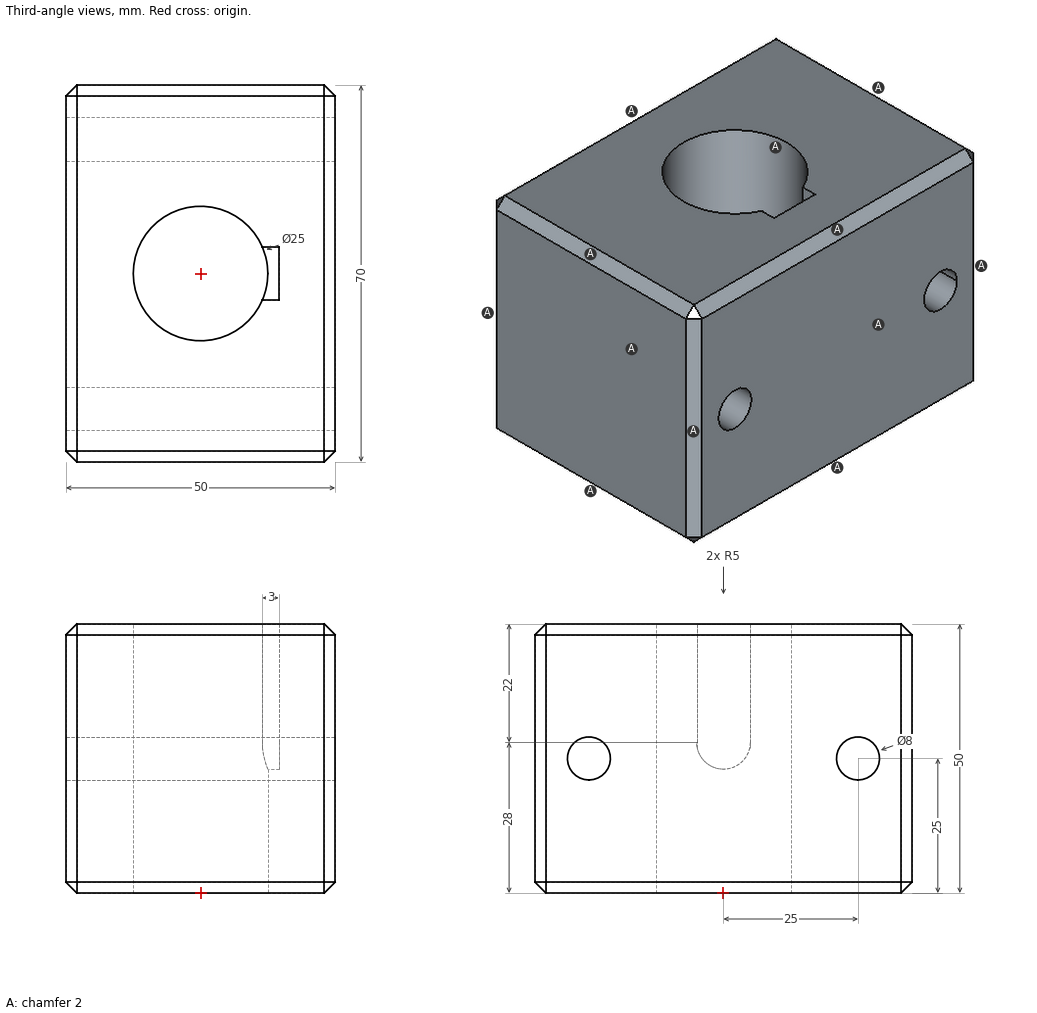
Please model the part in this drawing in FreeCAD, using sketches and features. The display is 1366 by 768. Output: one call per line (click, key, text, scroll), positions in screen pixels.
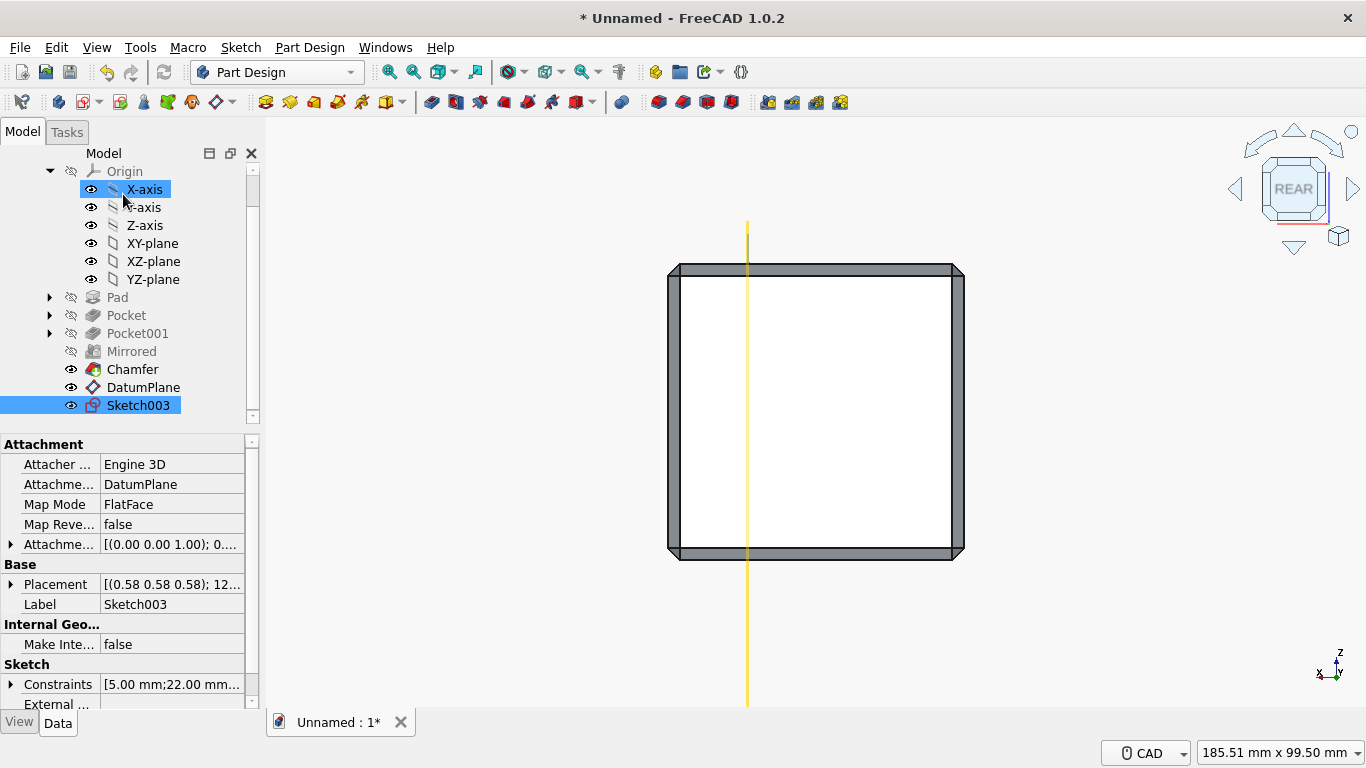
click(432, 102)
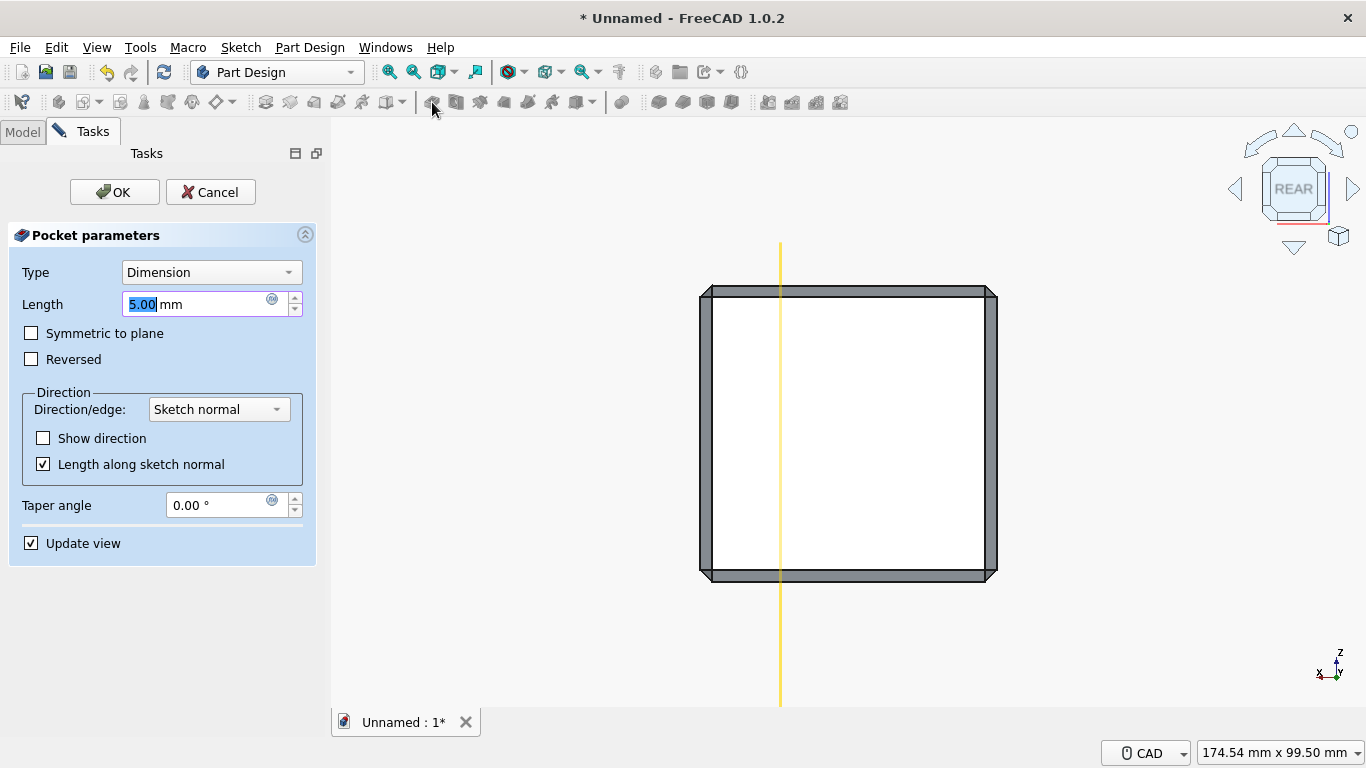
text(3)
key(Tab)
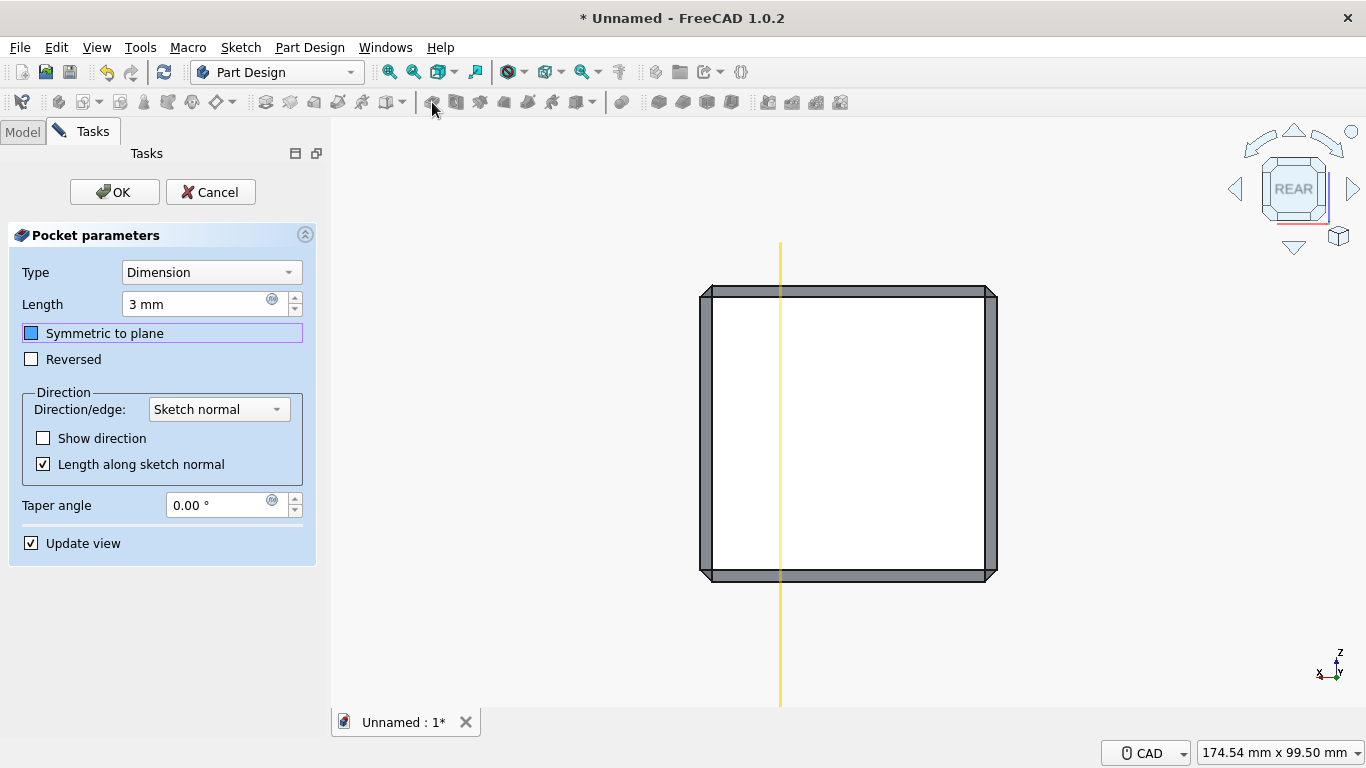
click(30, 359)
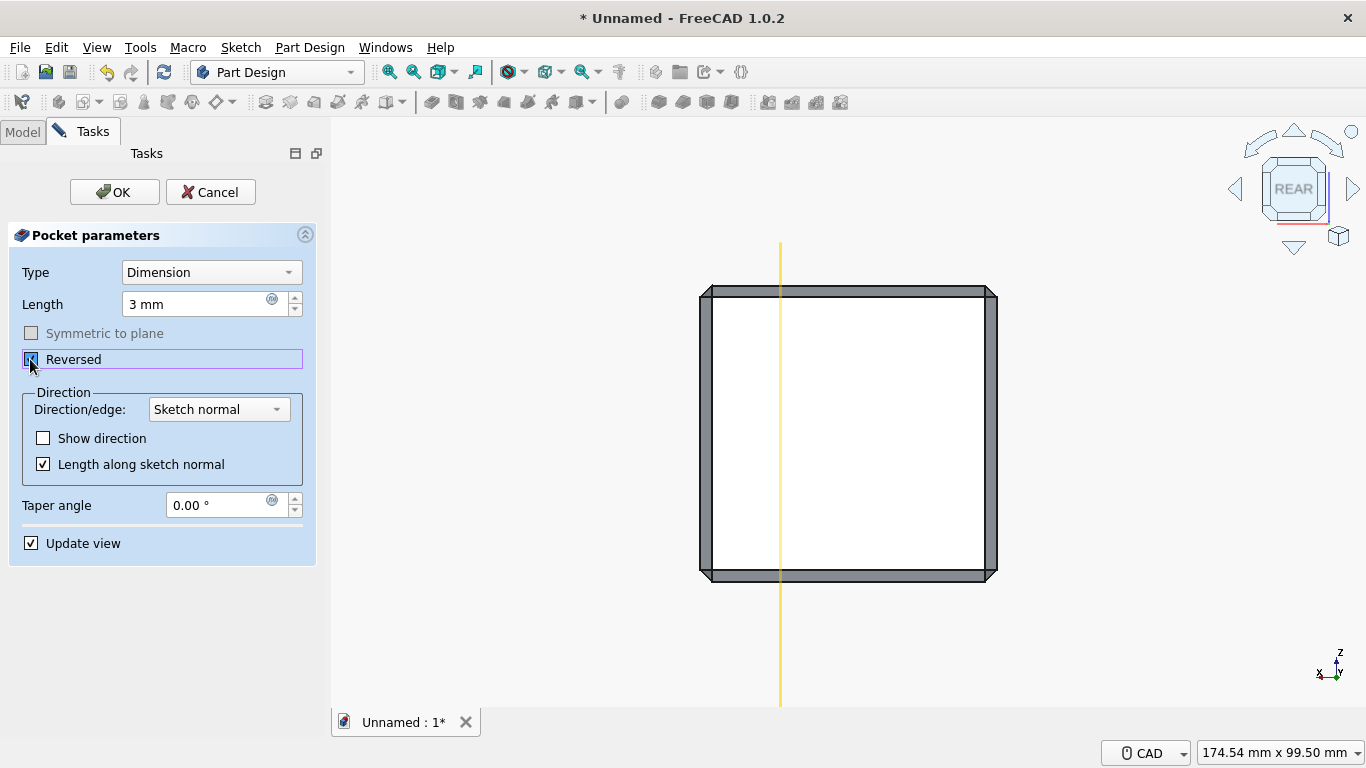
click(115, 192)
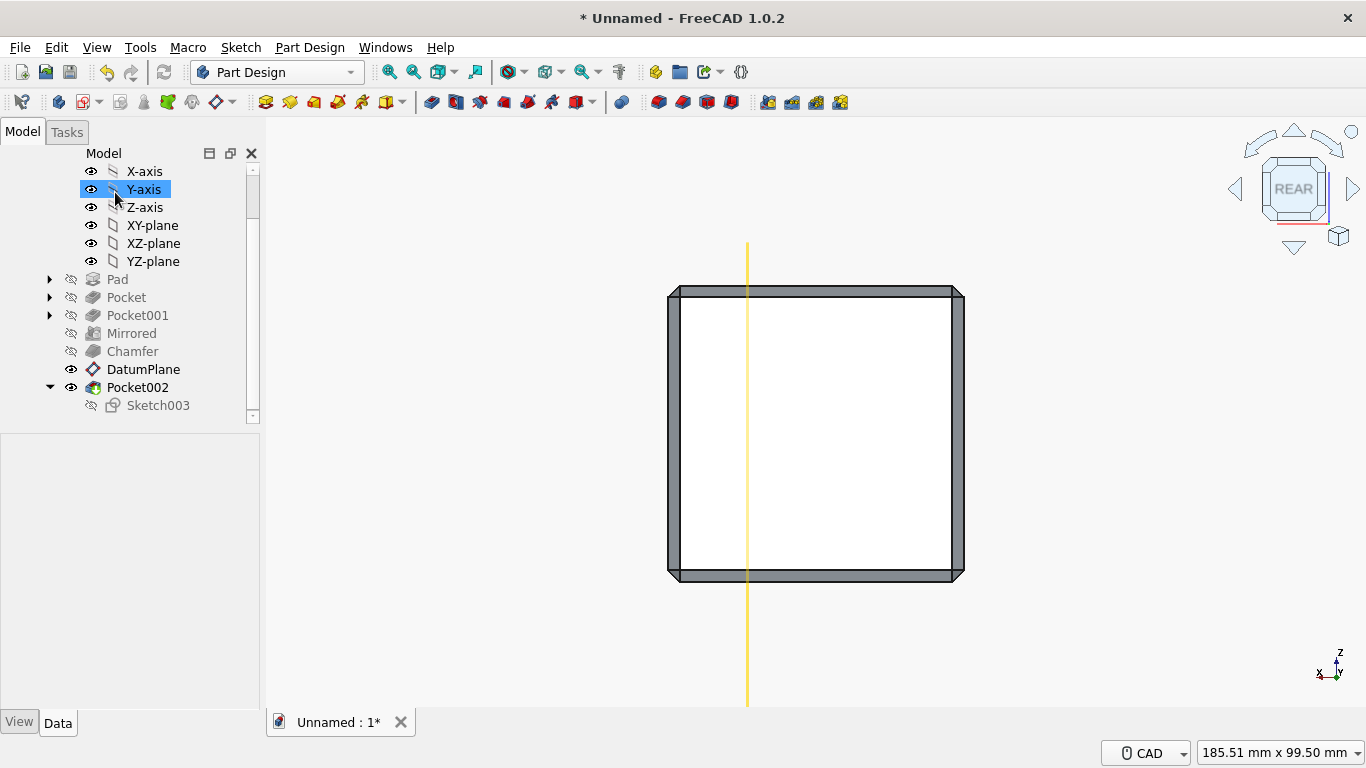
click(116, 369)
key(space)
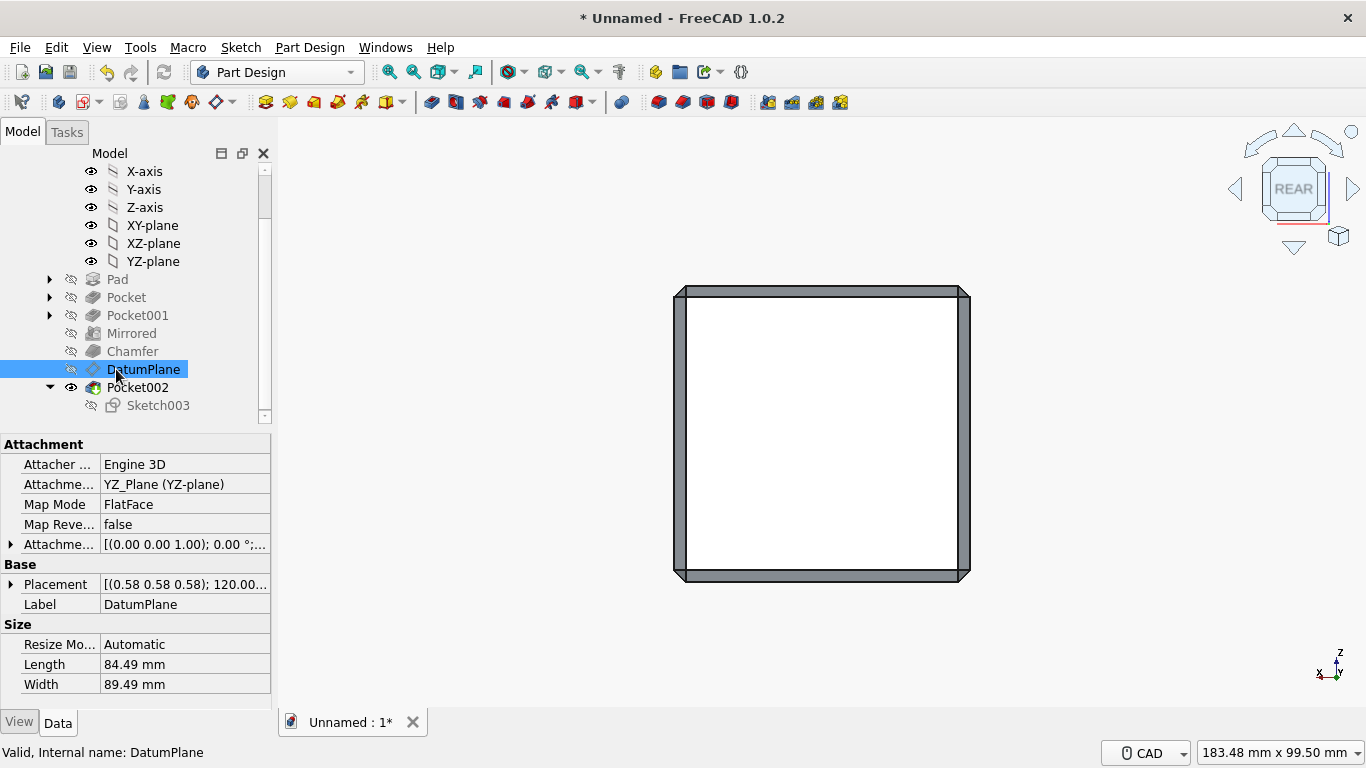
key(0)